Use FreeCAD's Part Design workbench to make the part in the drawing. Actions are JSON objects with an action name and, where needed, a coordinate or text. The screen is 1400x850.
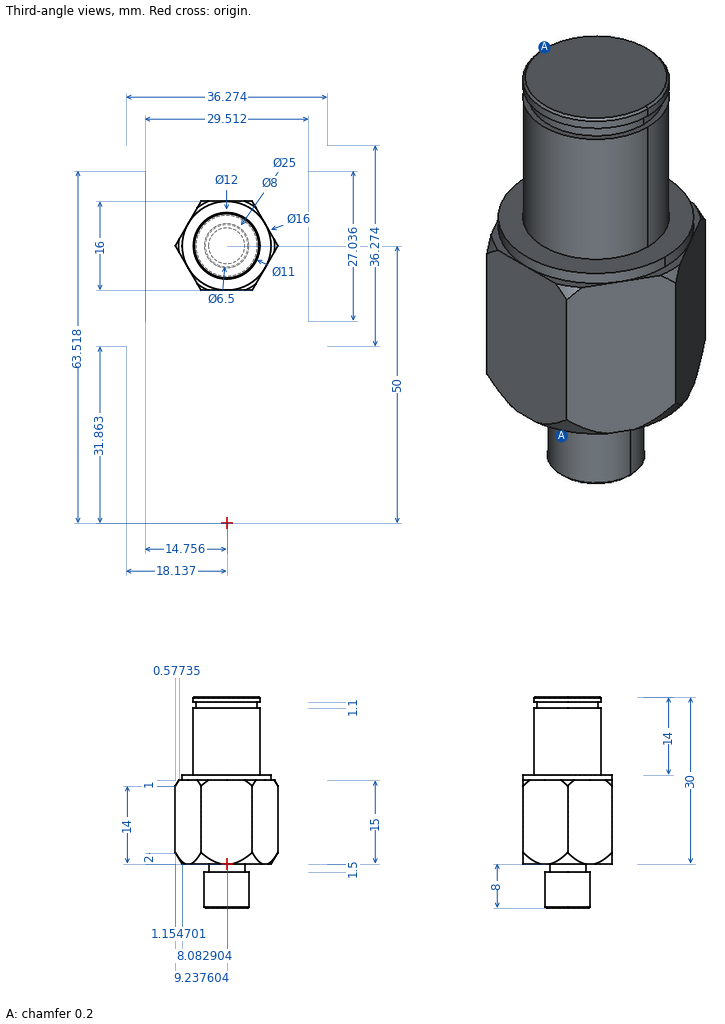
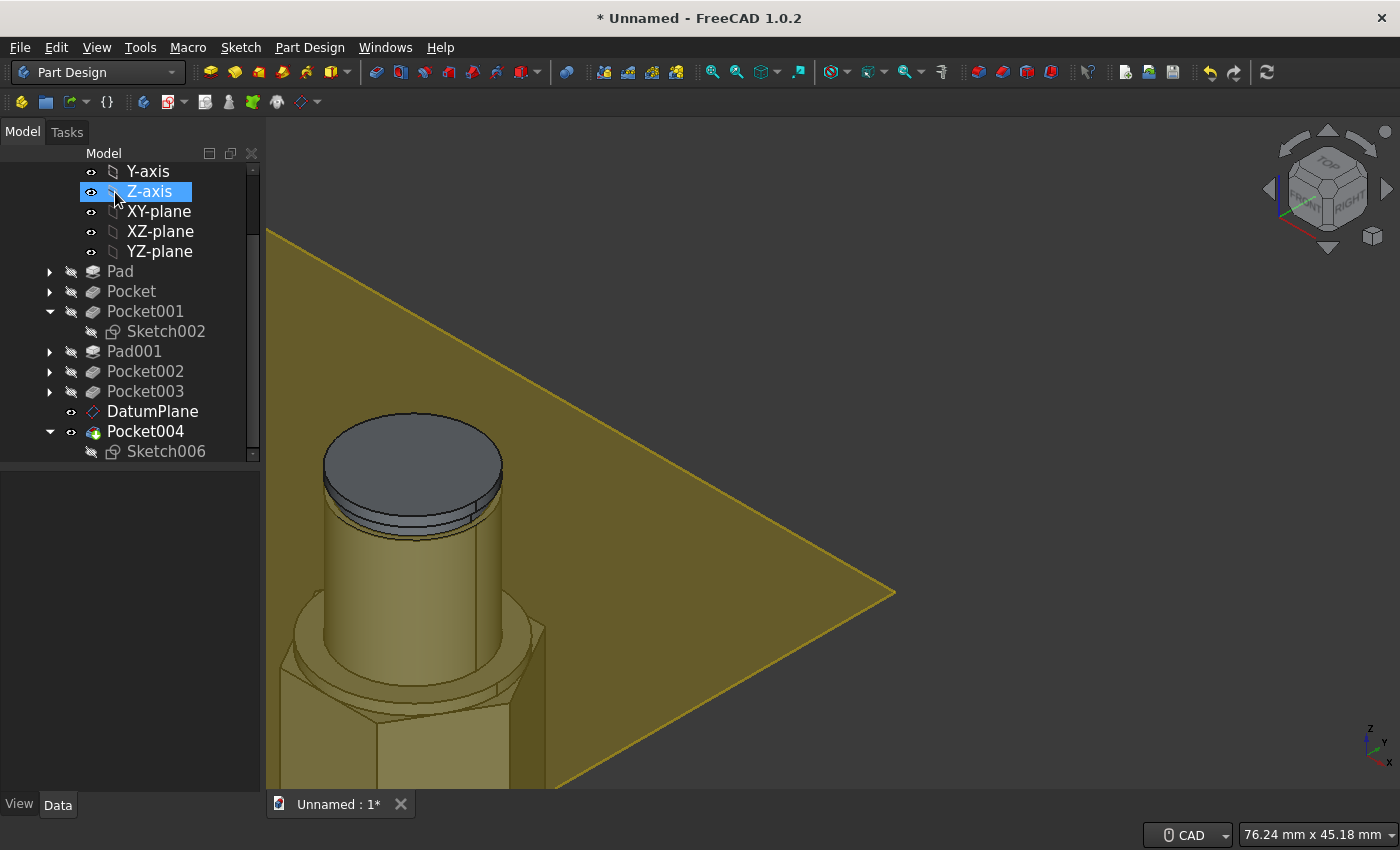
{"action": "left_click", "coordinate": [116, 412]}
{"action": "key", "text": "space"}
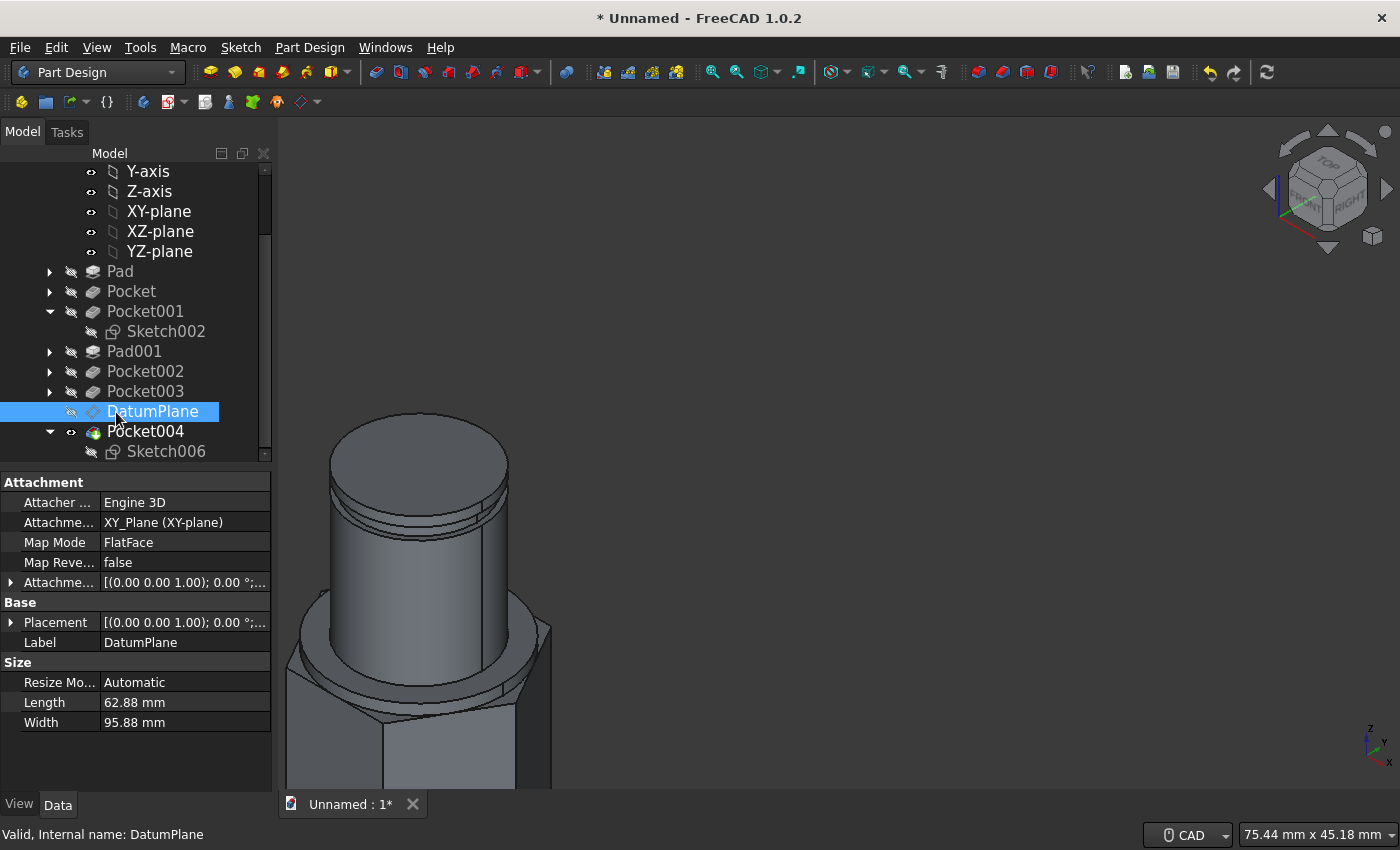
{"action": "left_click", "coordinate": [714, 72]}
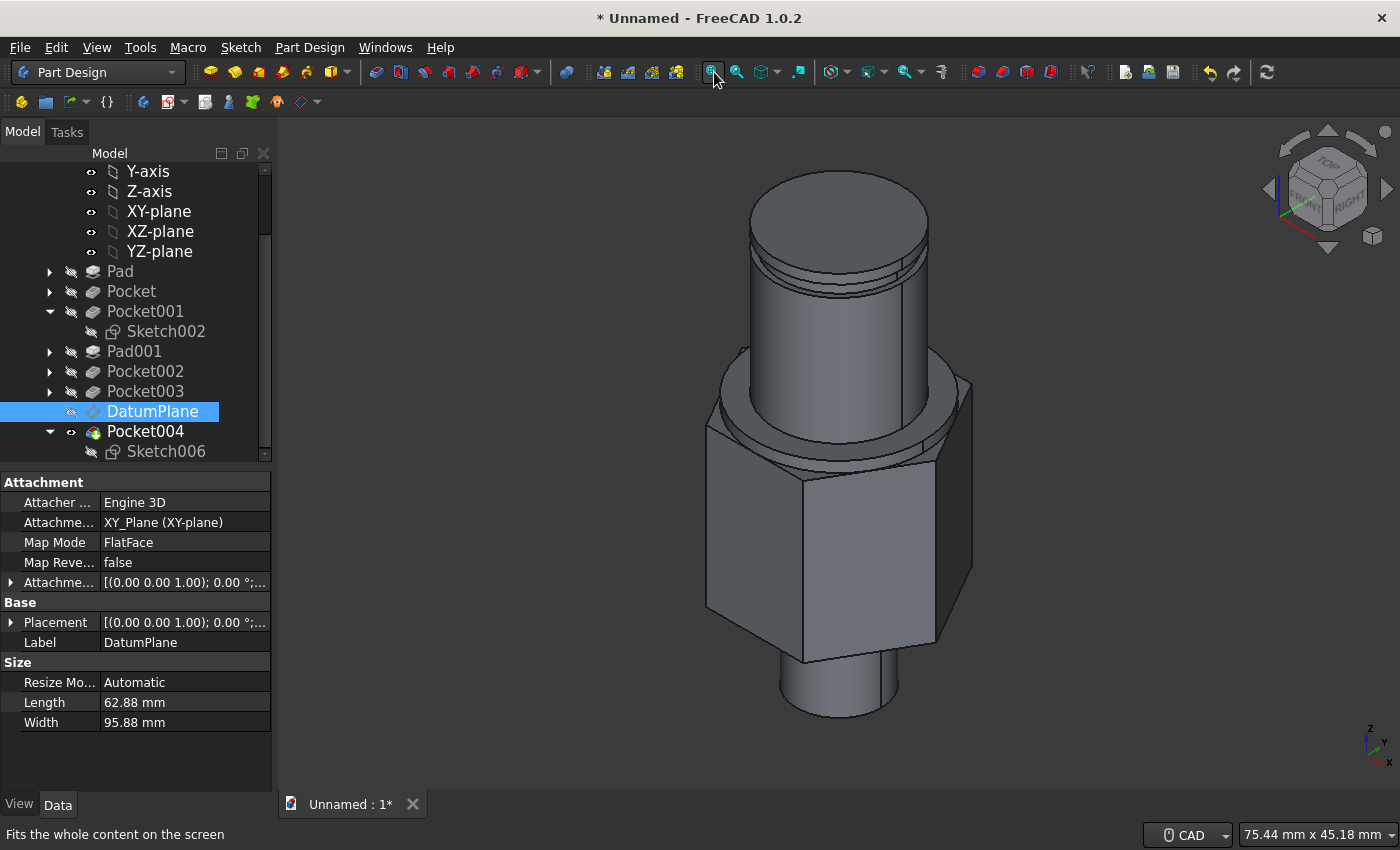
{"action": "left_click", "coordinate": [759, 245]}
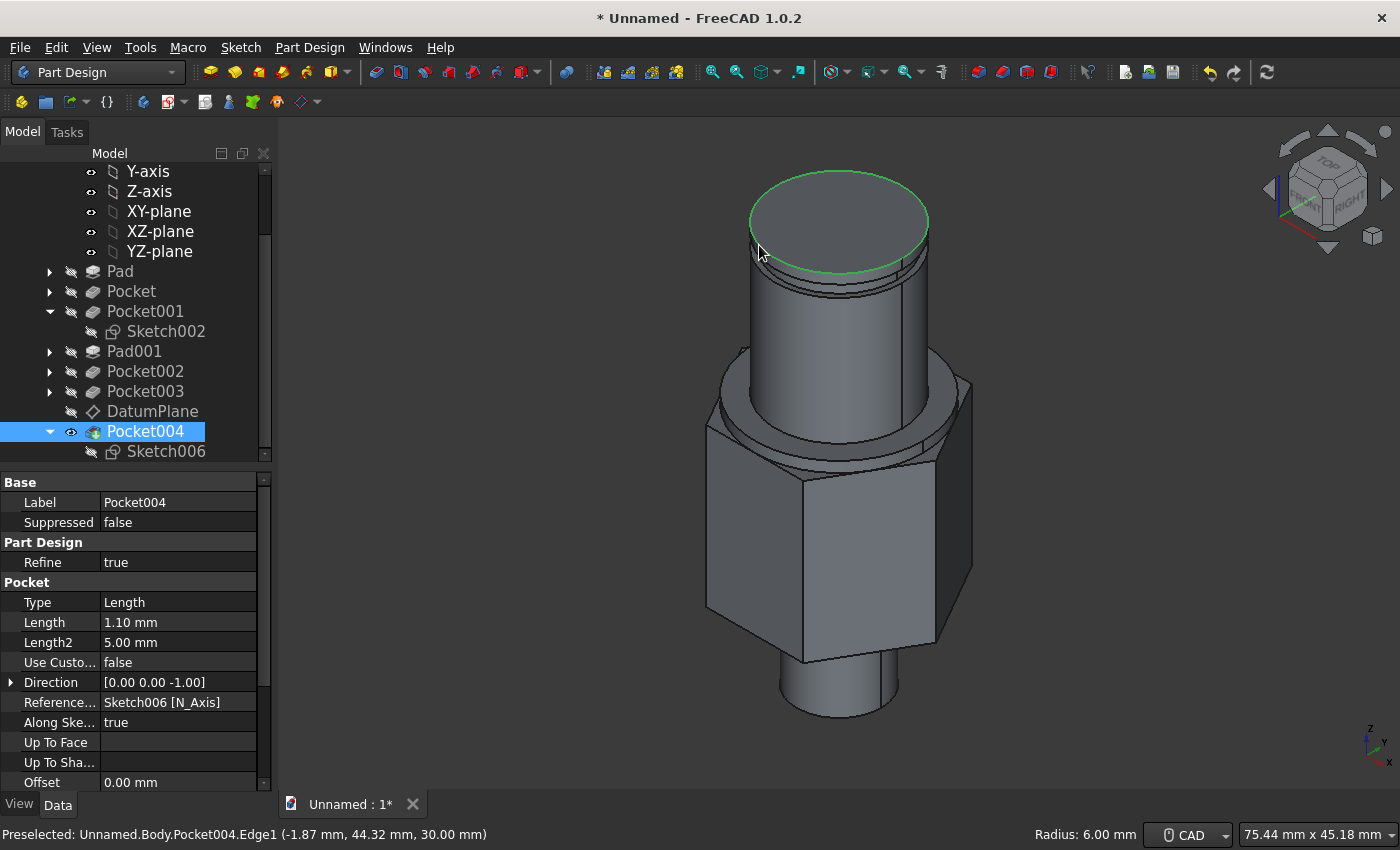
{"action": "key", "text": "2"}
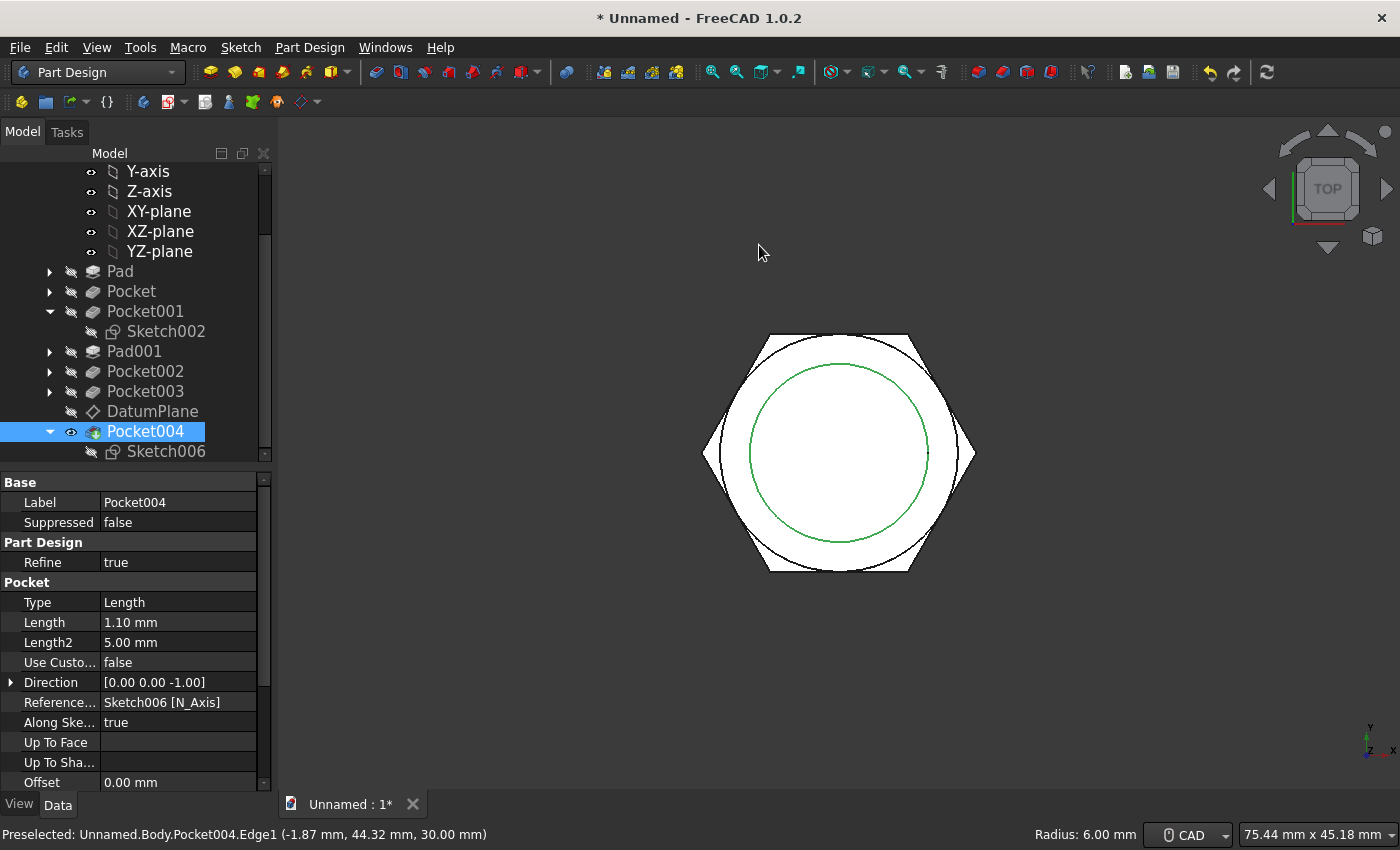
{"action": "left_click", "coordinate": [714, 72]}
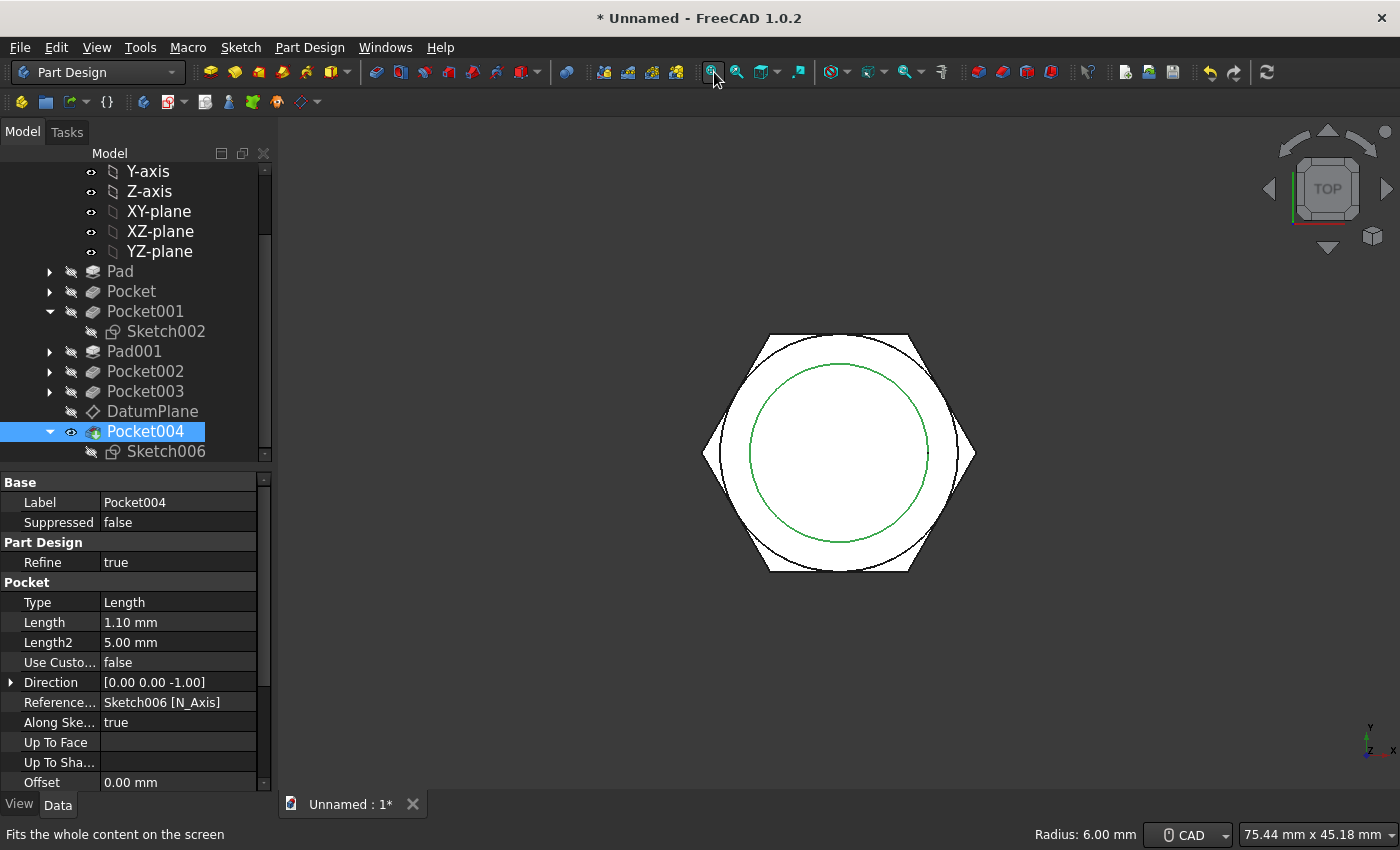
{"action": "key", "text": "0"}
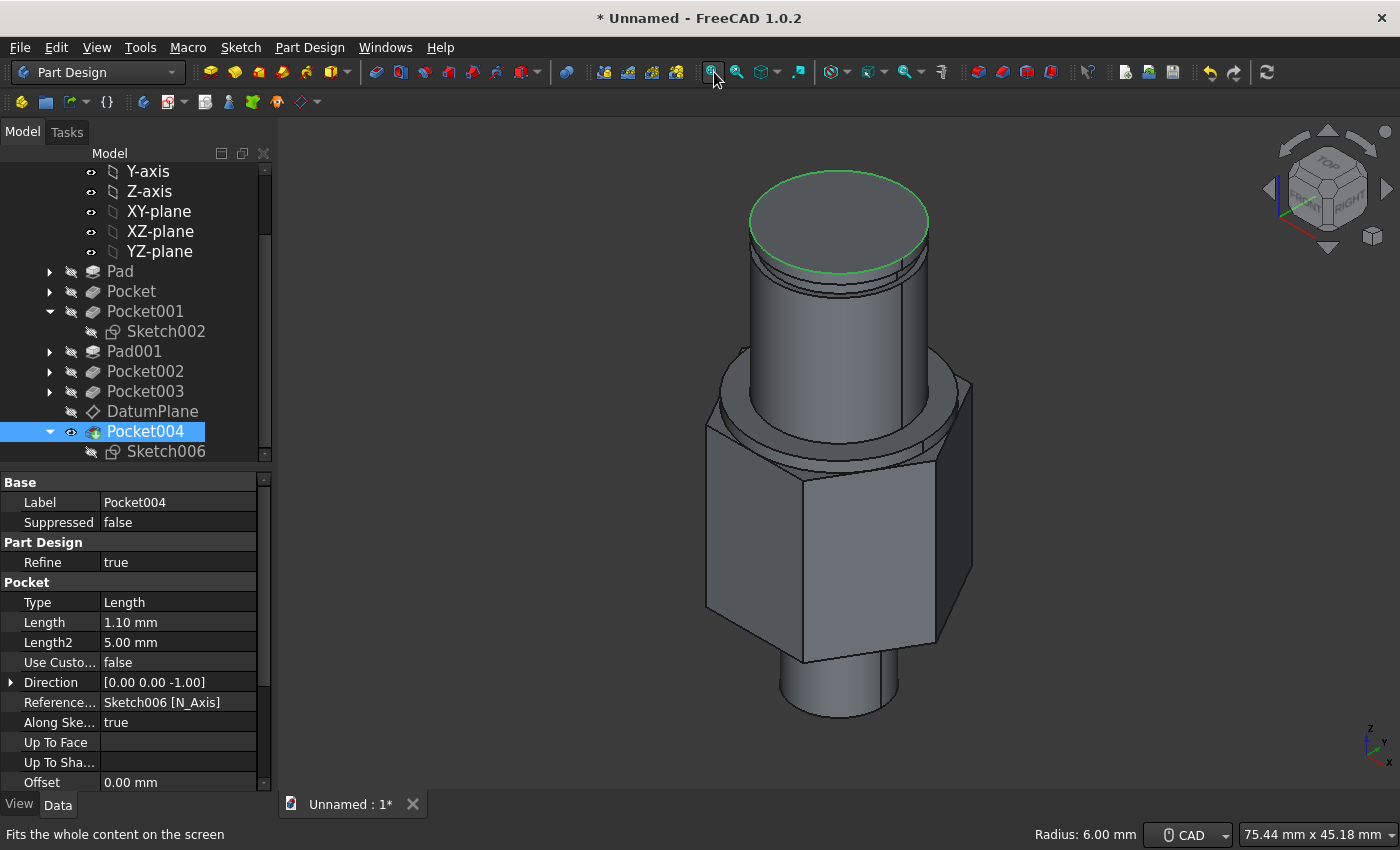
{"action": "key", "text": "1"}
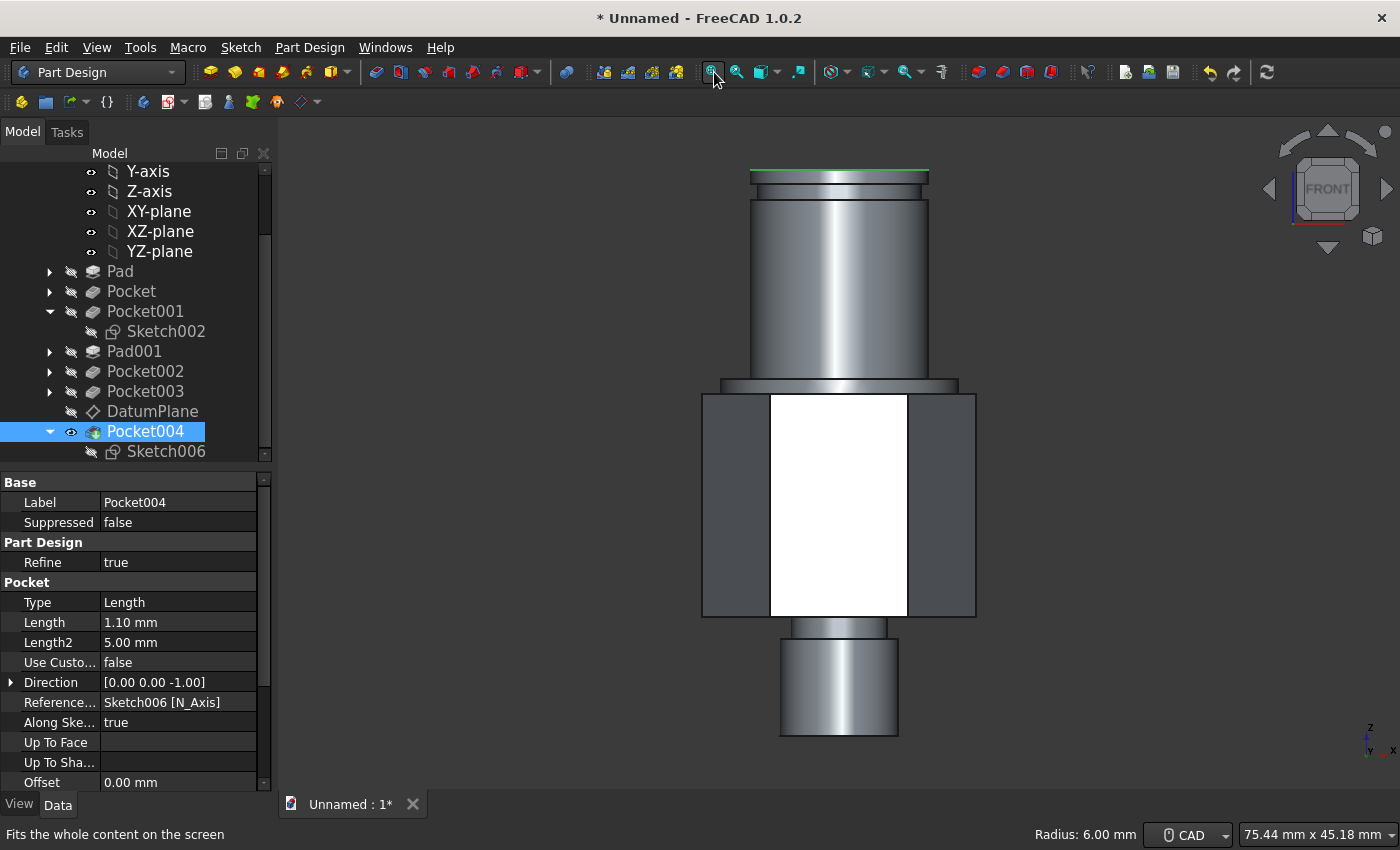
{"action": "left_click", "coordinate": [780, 735], "text": "ctrl"}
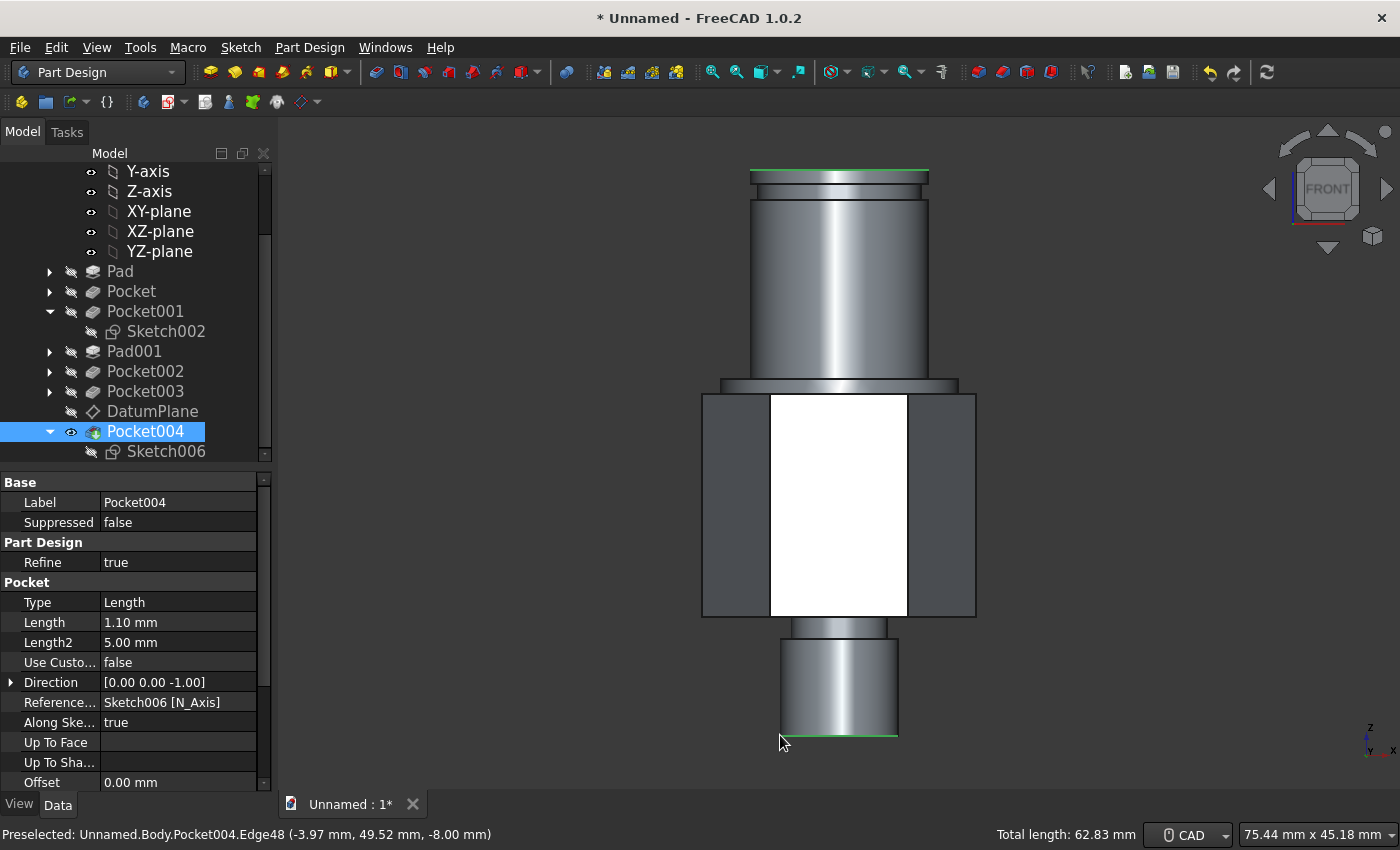
{"action": "left_click", "coordinate": [1004, 72]}